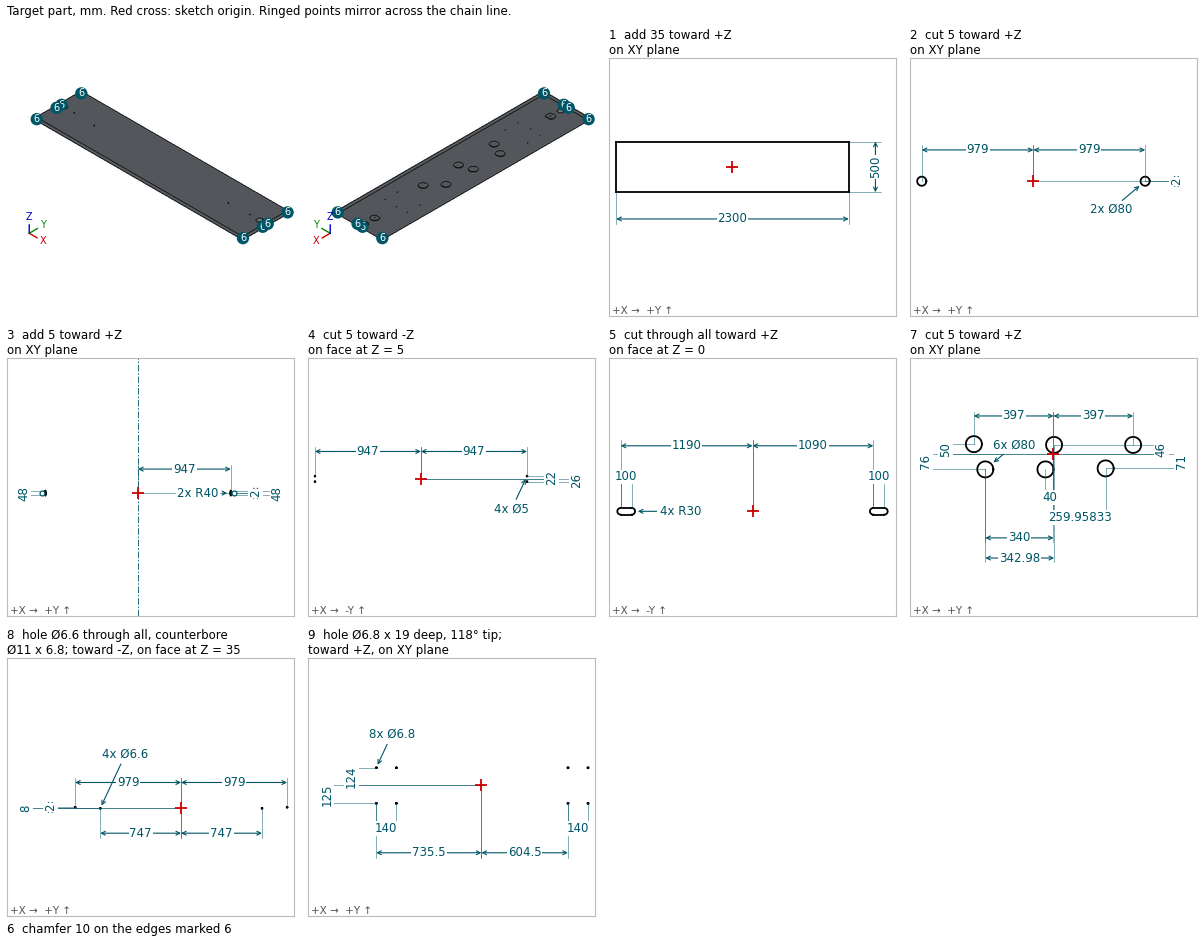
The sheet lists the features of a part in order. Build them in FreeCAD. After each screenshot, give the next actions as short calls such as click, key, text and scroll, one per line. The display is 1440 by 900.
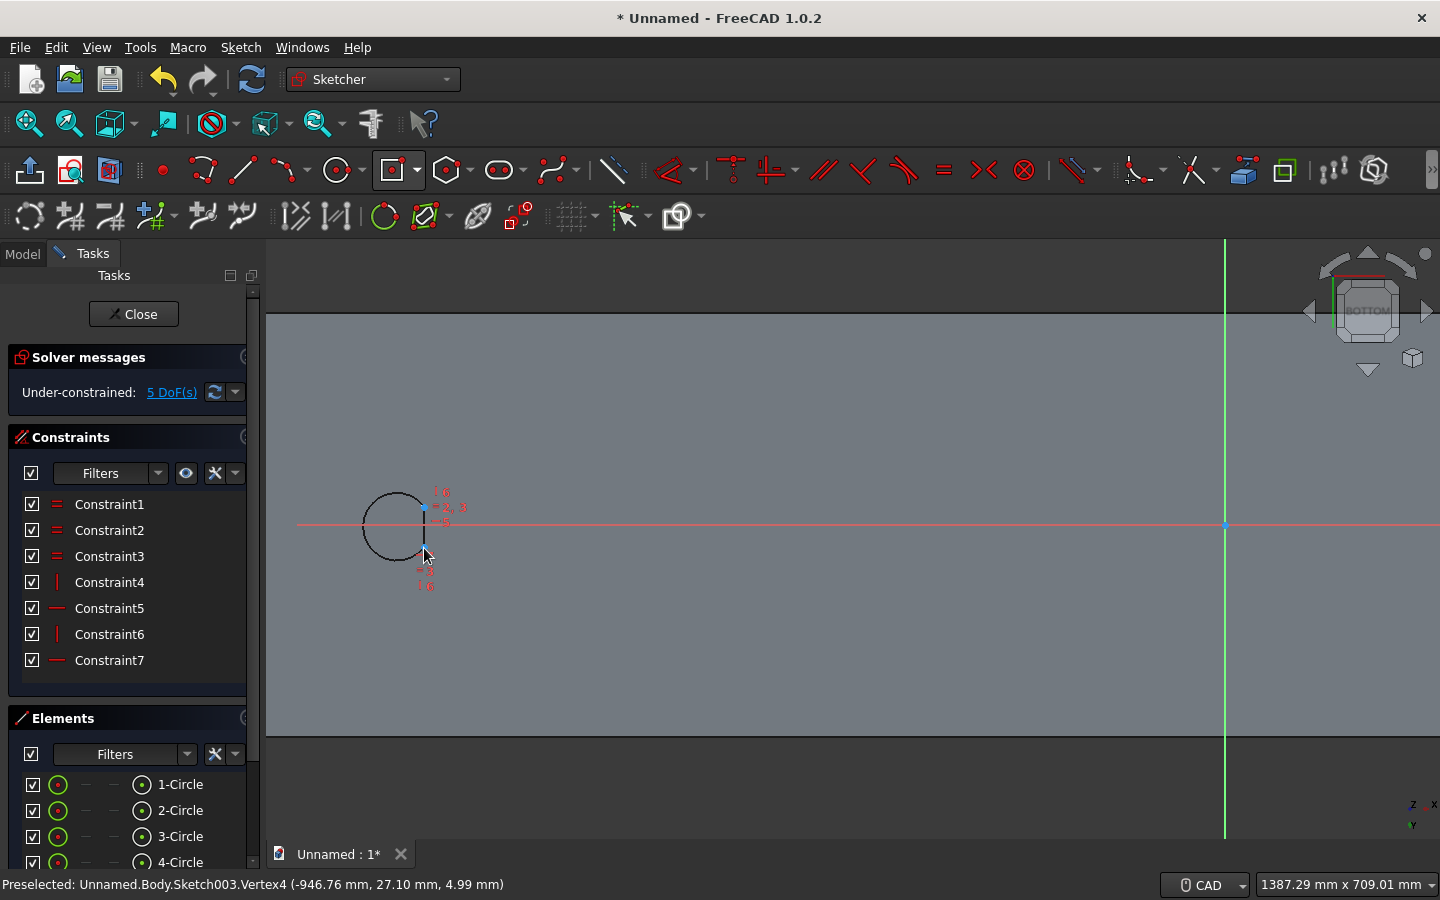
click(668, 170)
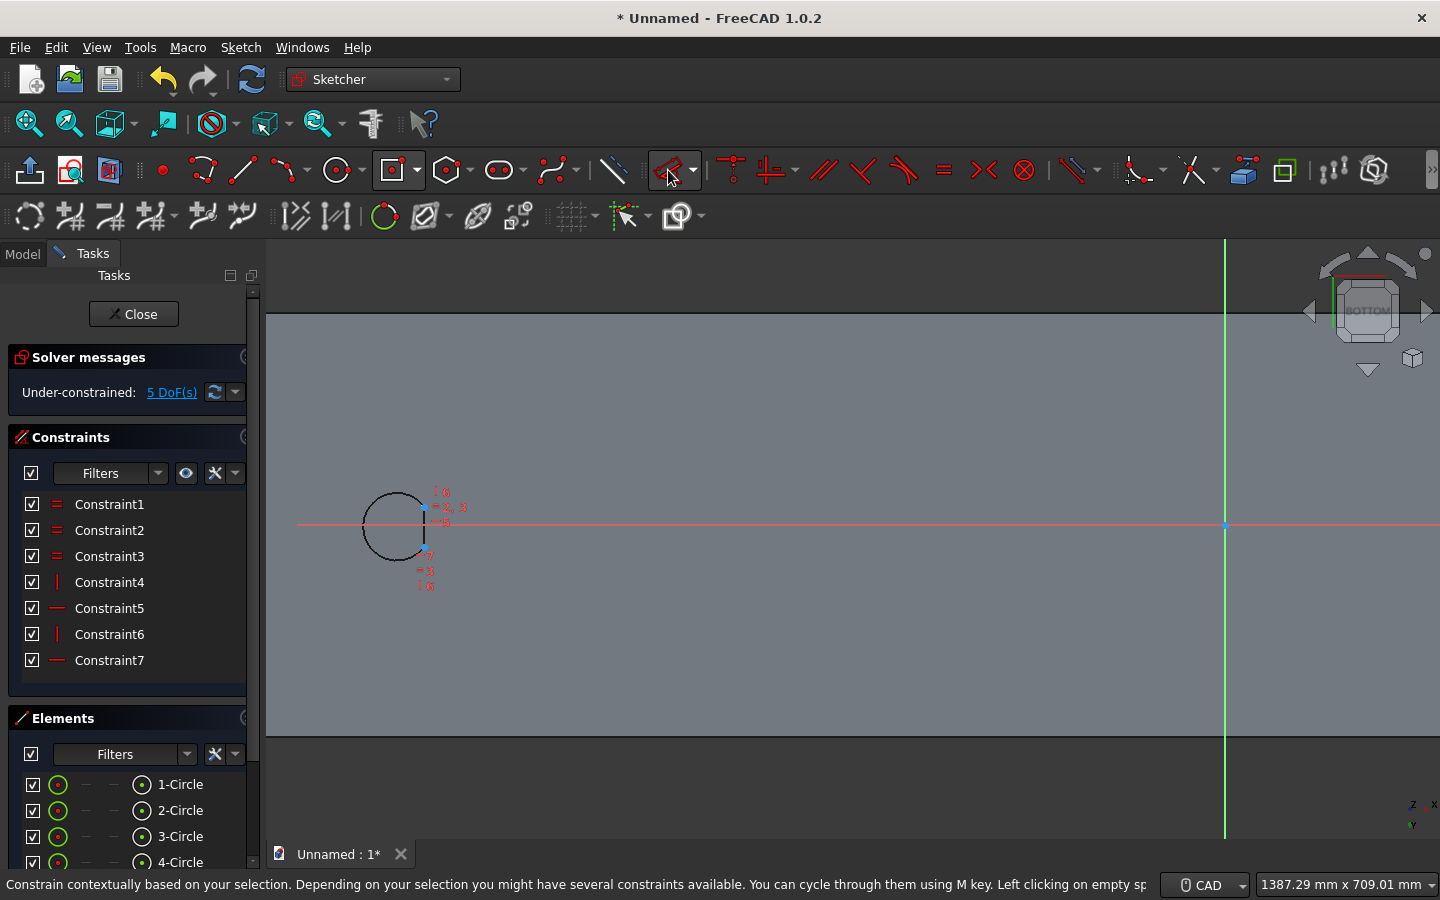
scroll(425, 549, down, 4)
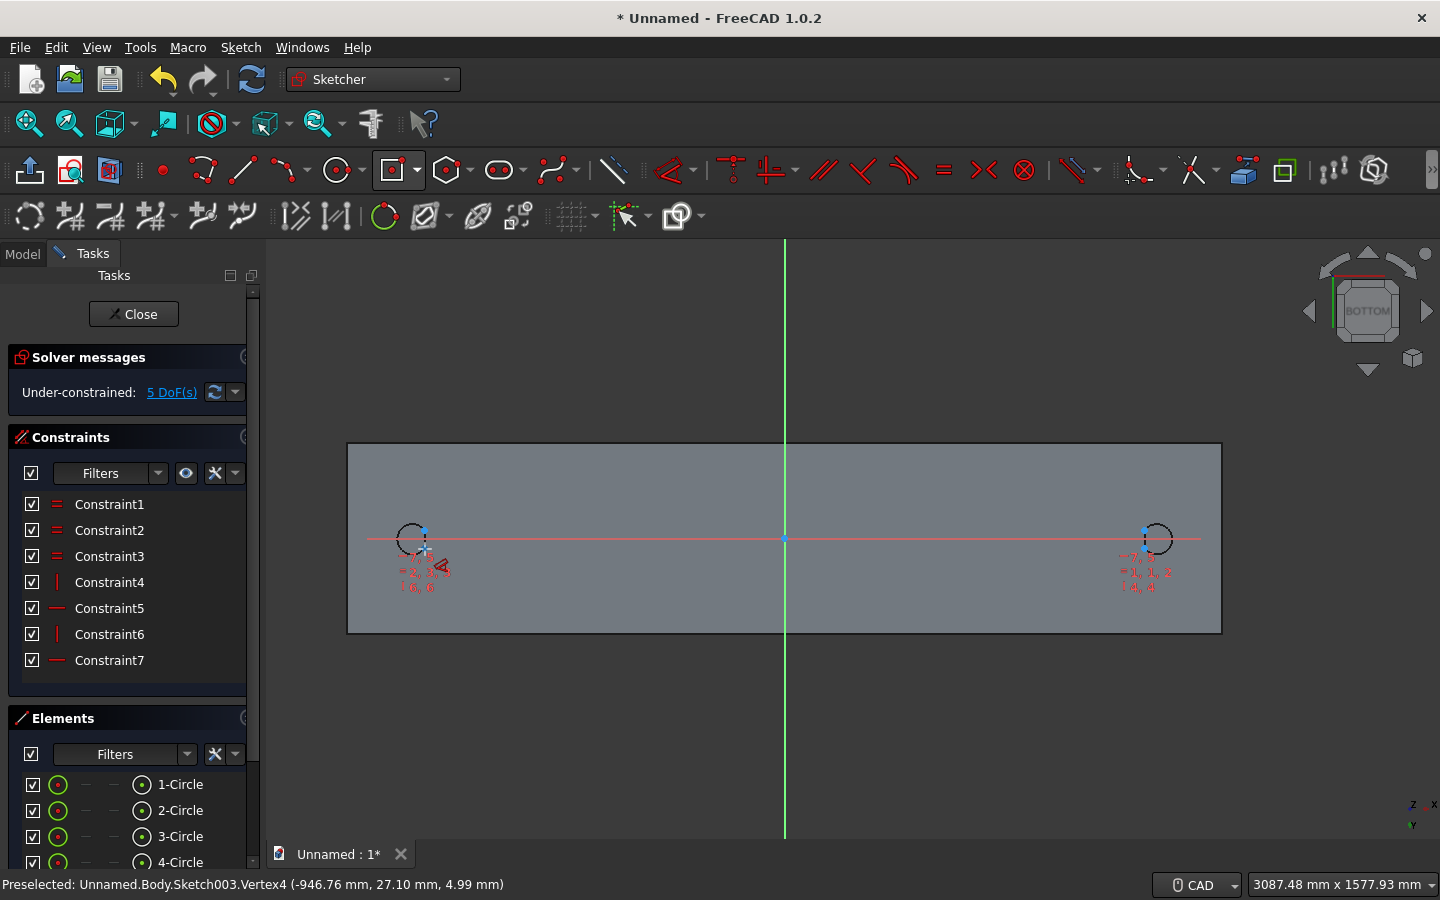
scroll(1145, 529, up, 16)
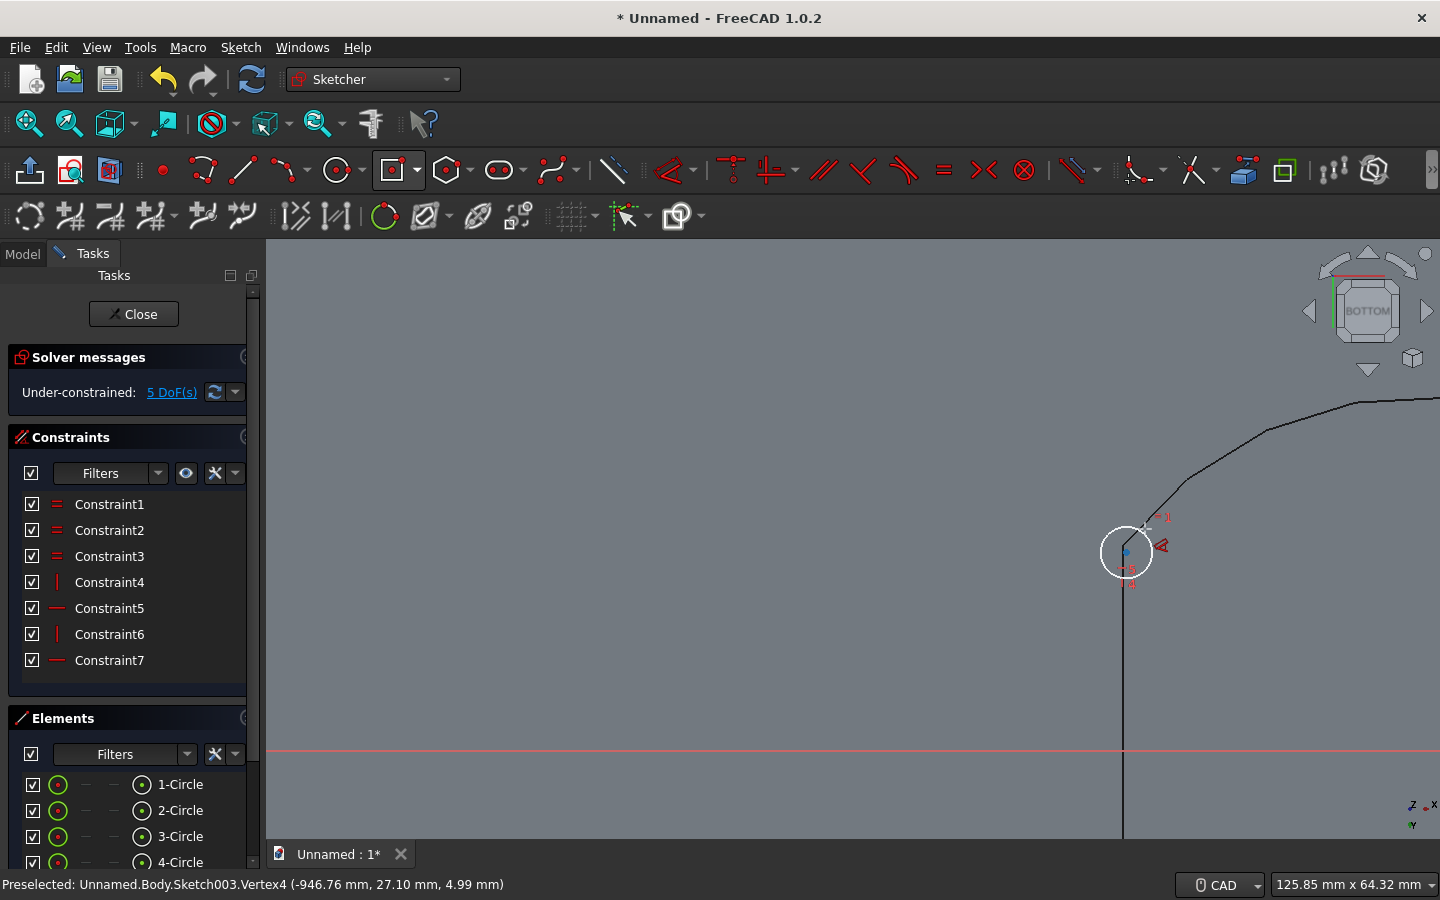
click(1127, 527)
click(1128, 495)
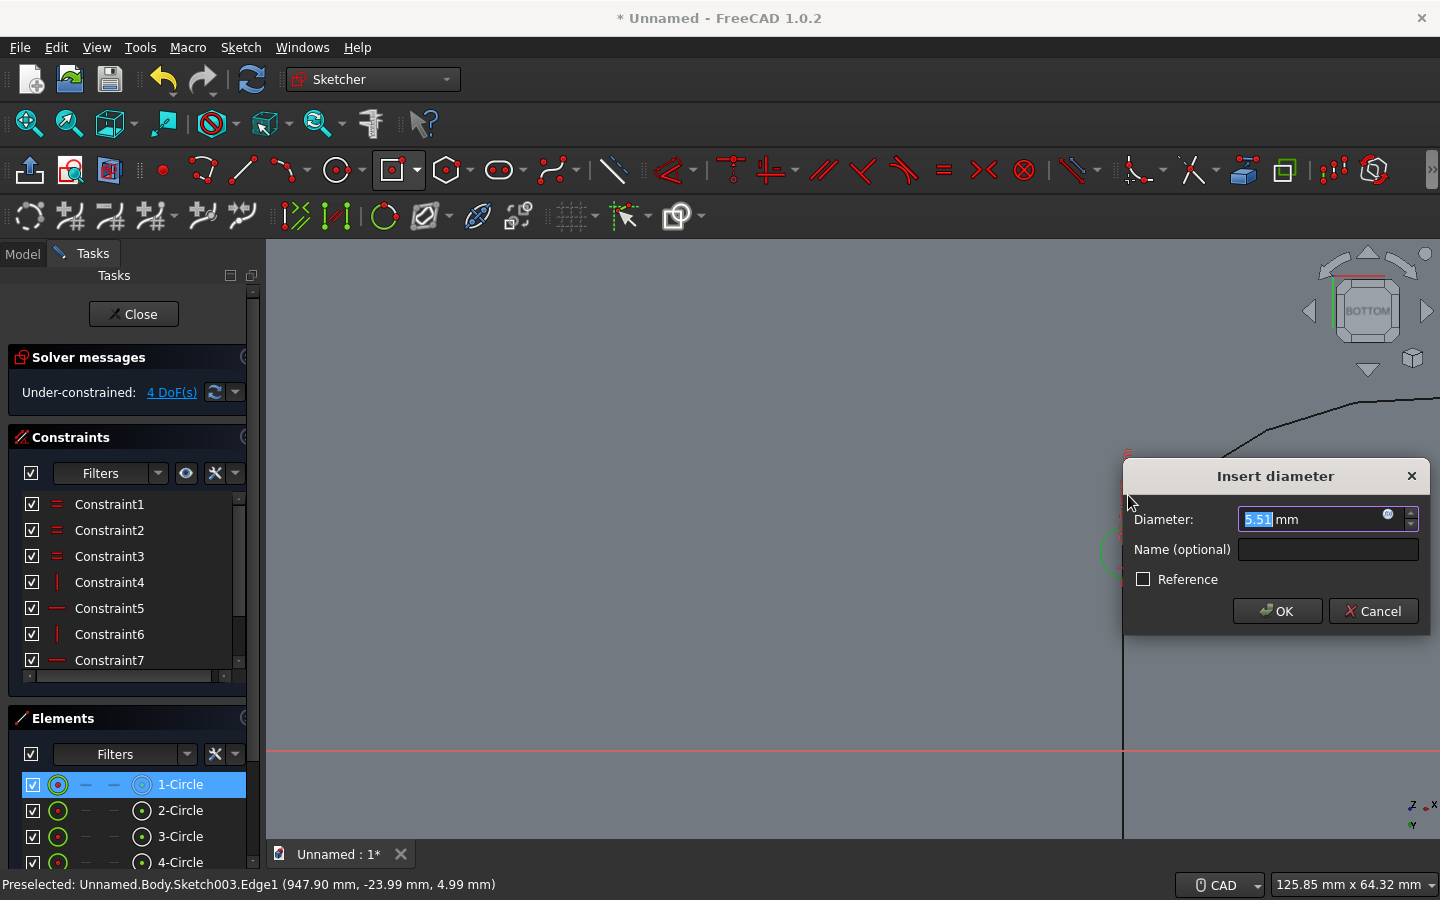
text(5)
key(Return)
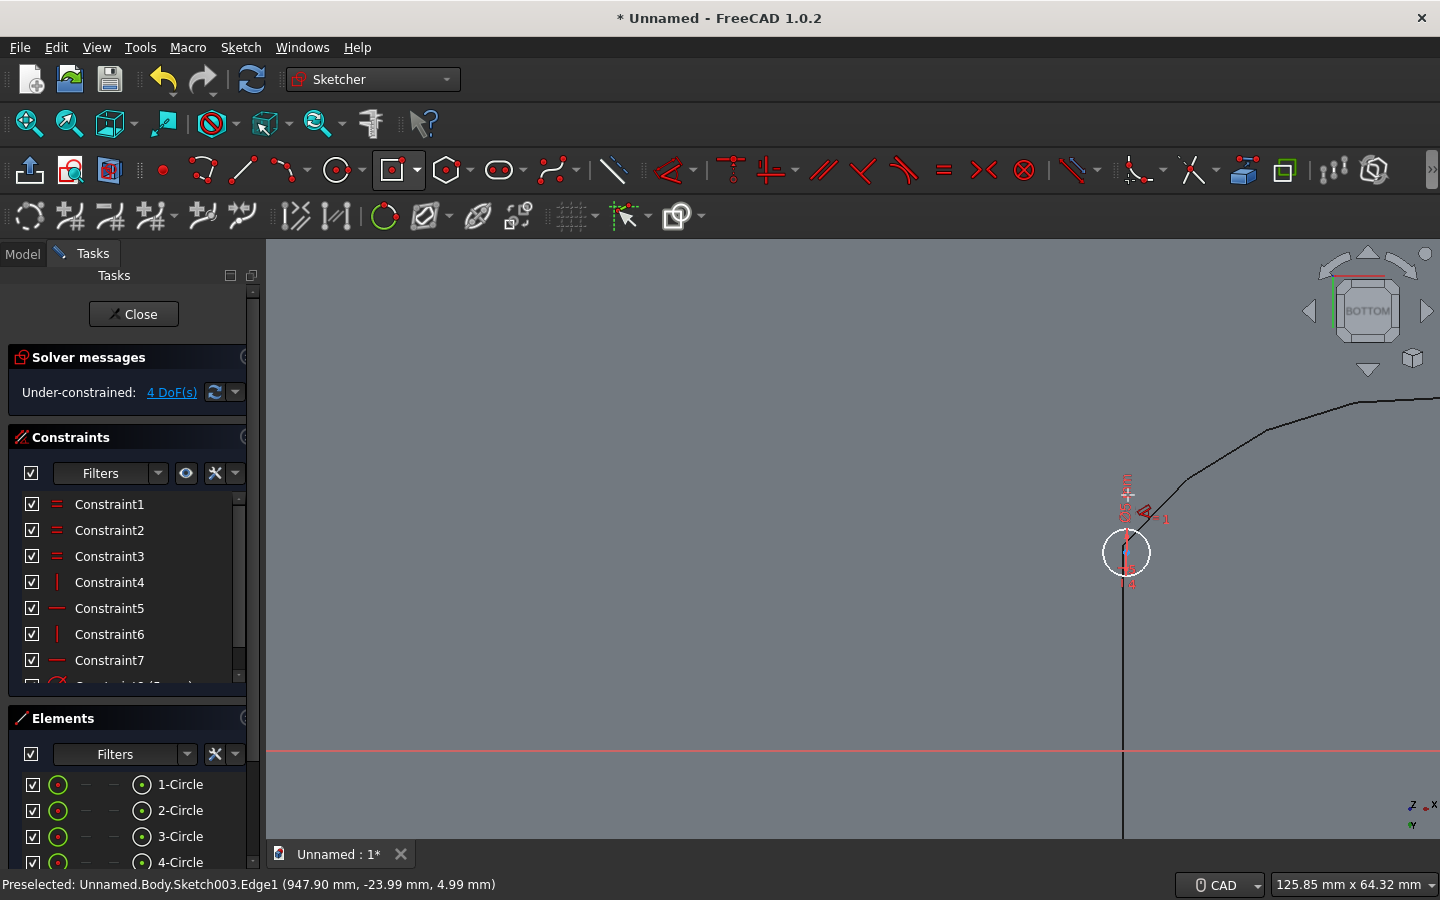
scroll(1230, 527, down, 15)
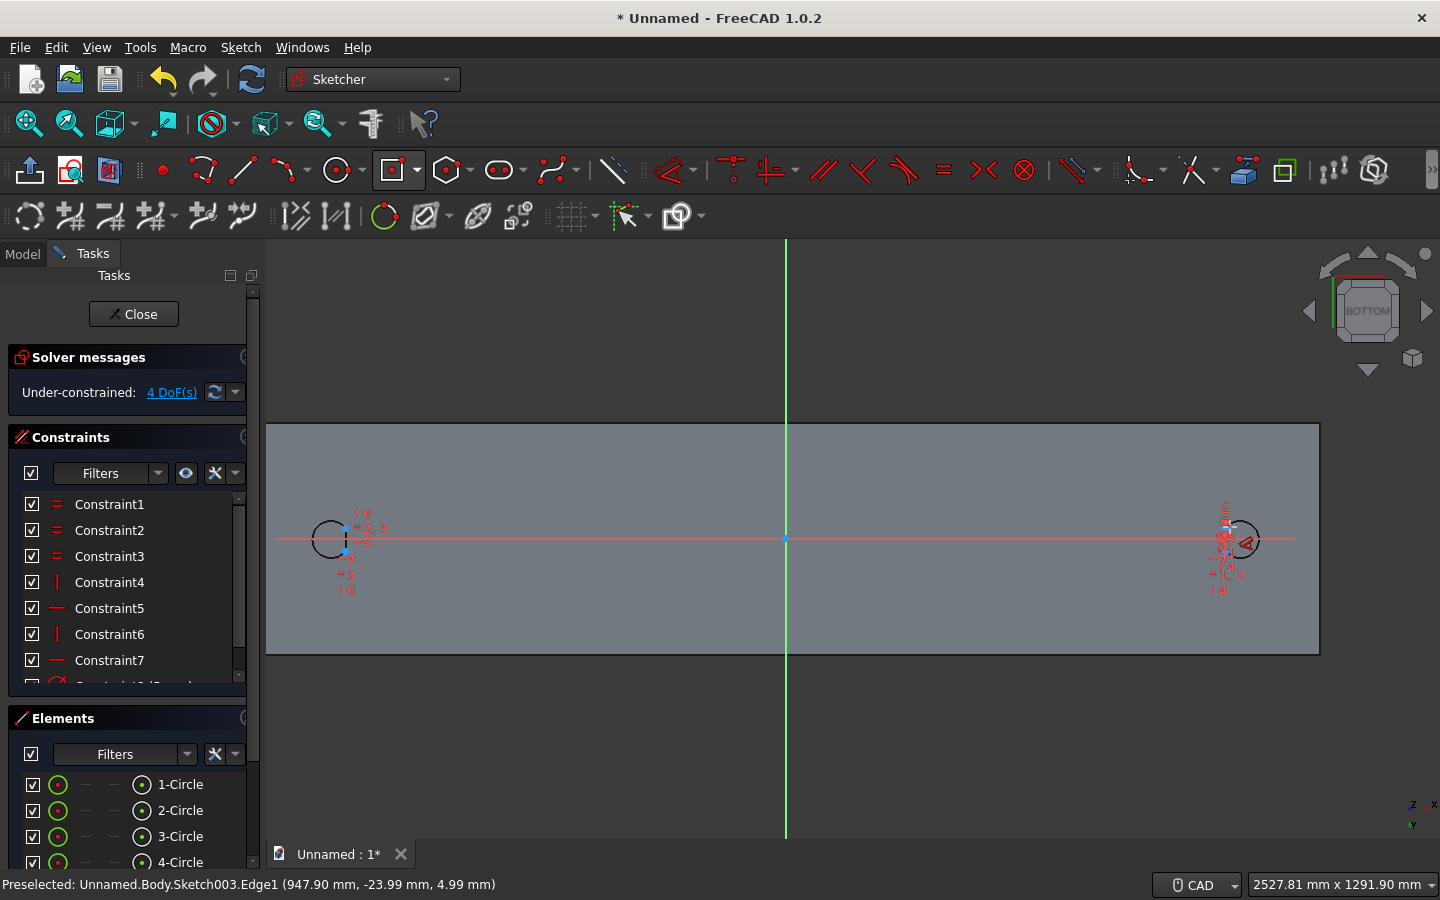
scroll(1226, 529, up, 7)